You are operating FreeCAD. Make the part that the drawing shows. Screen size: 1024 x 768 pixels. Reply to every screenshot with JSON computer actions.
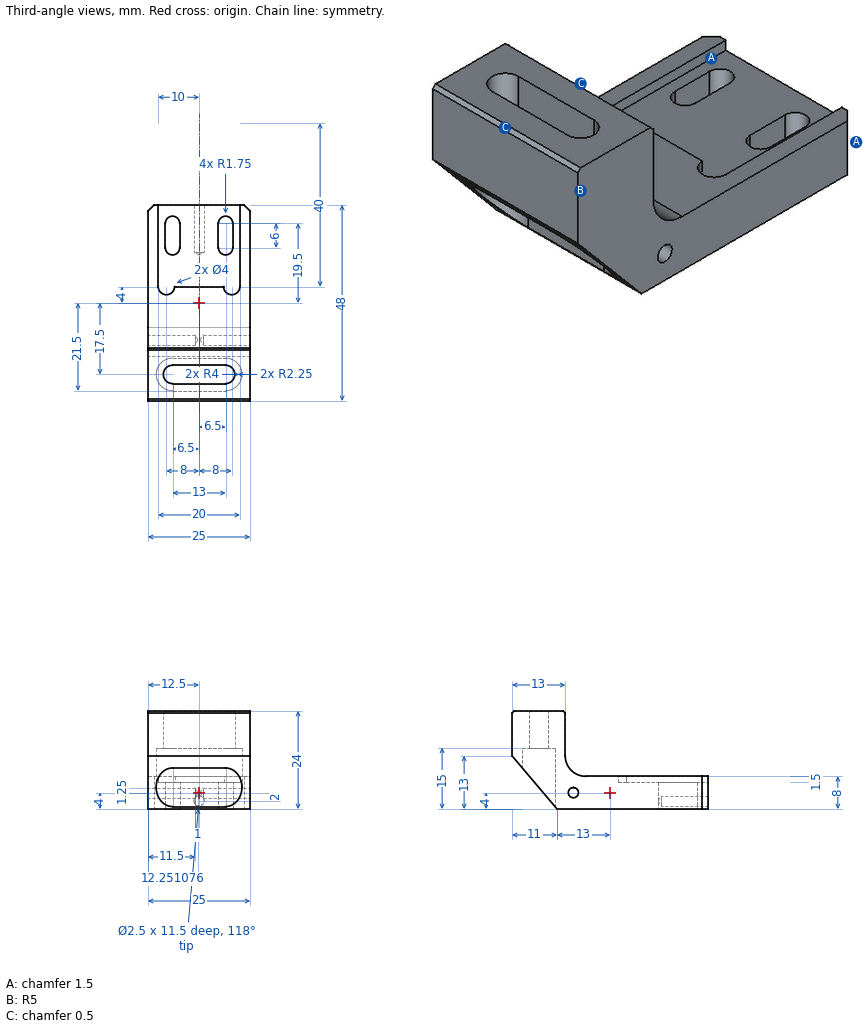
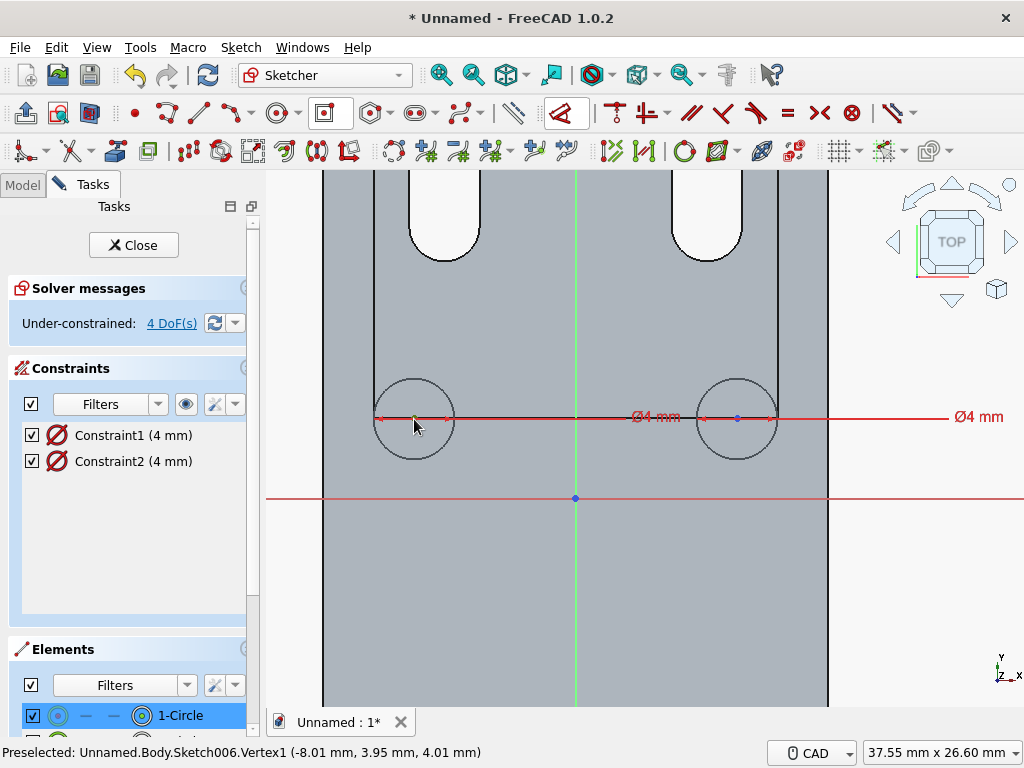
{"action": "left_click", "coordinate": [737, 419]}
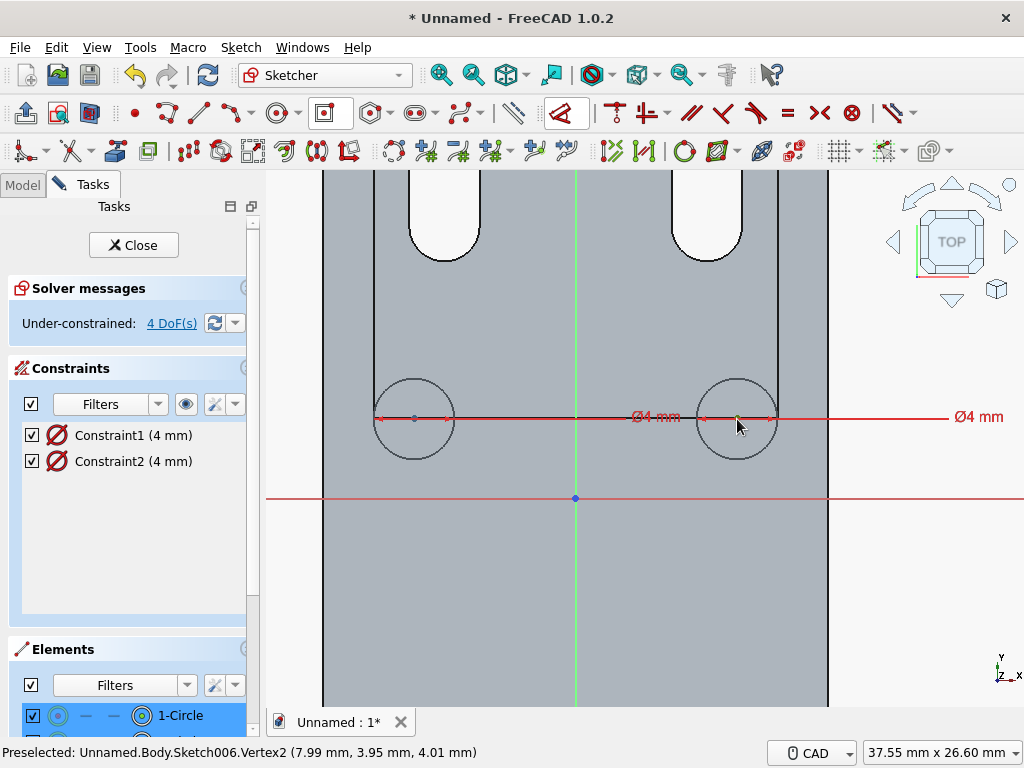
{"action": "left_click", "coordinate": [670, 114]}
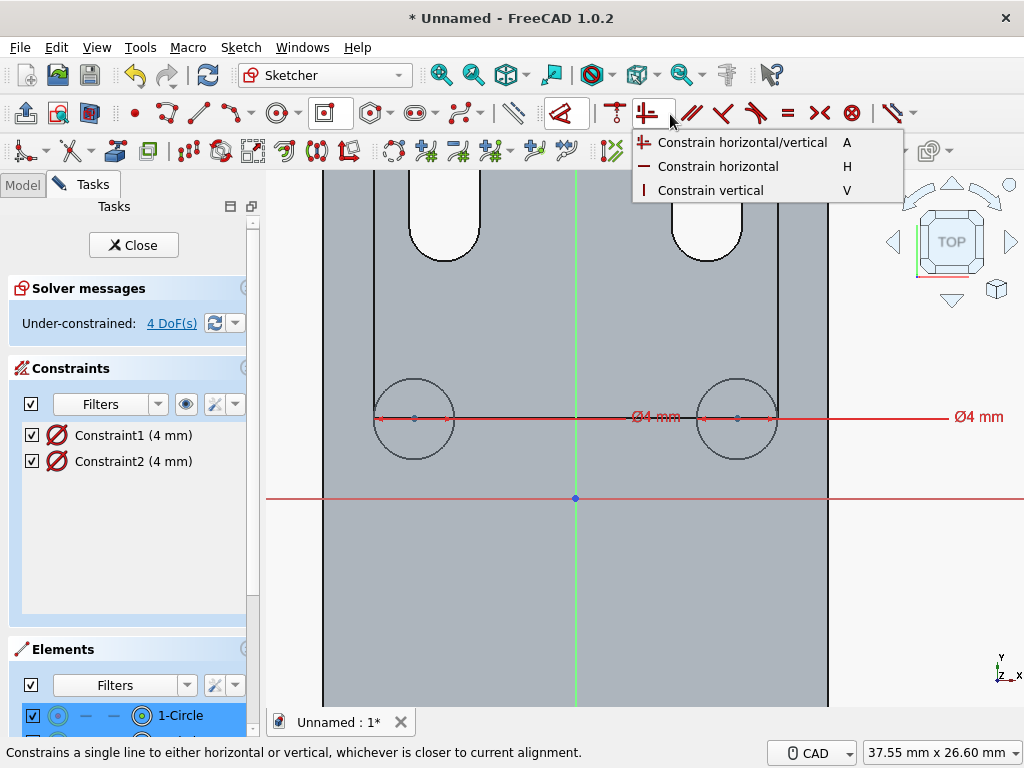
{"action": "left_click", "coordinate": [768, 166]}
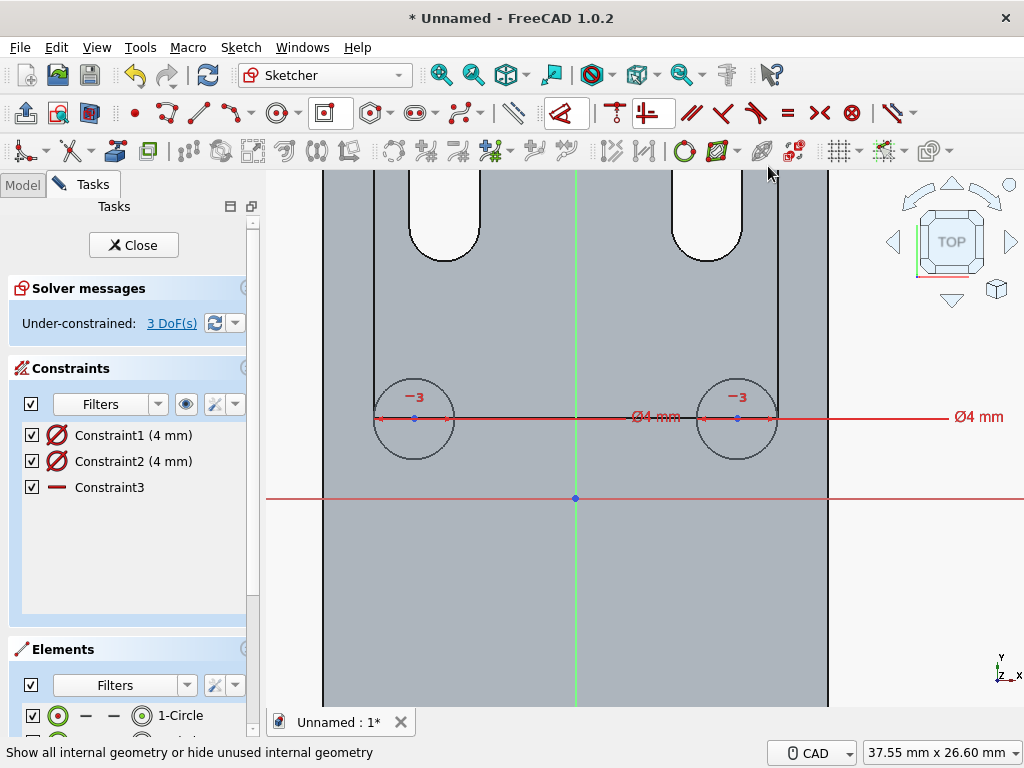
{"action": "left_click", "coordinate": [414, 419]}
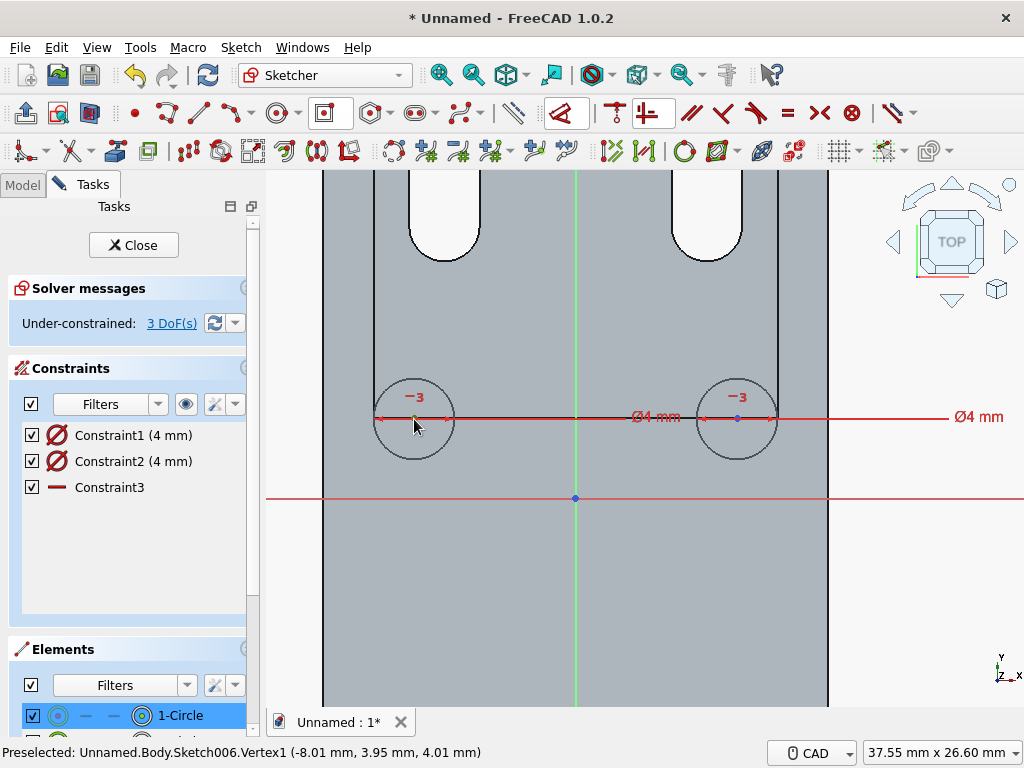
{"action": "left_click", "coordinate": [584, 114]}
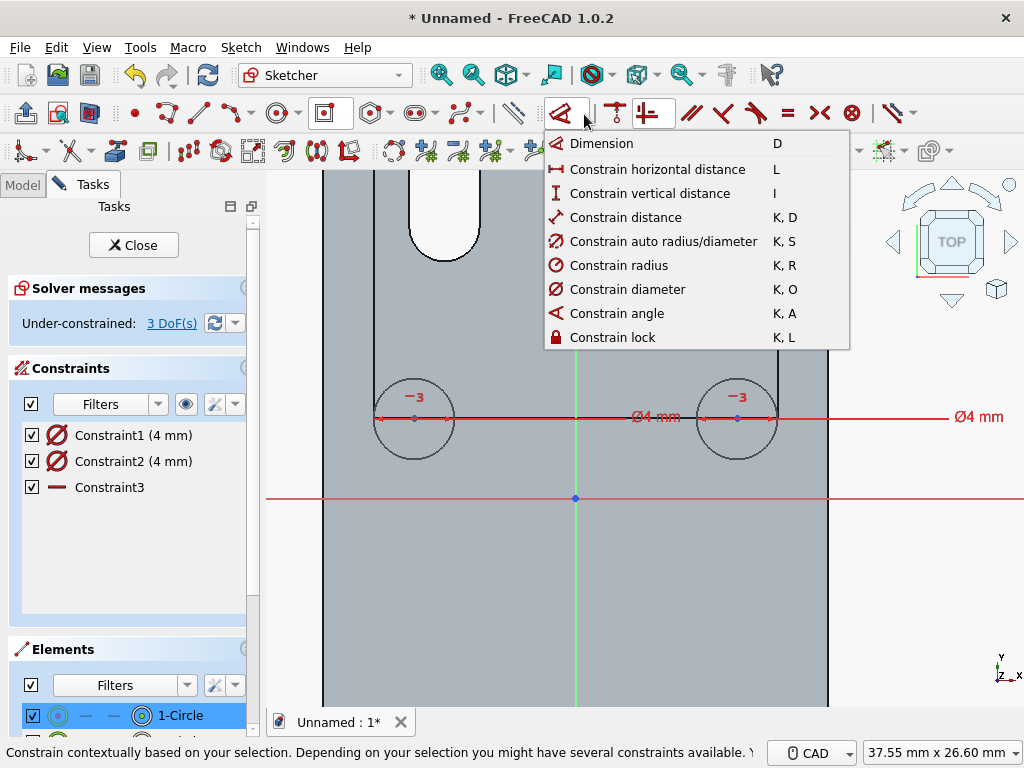
{"action": "left_click", "coordinate": [697, 169]}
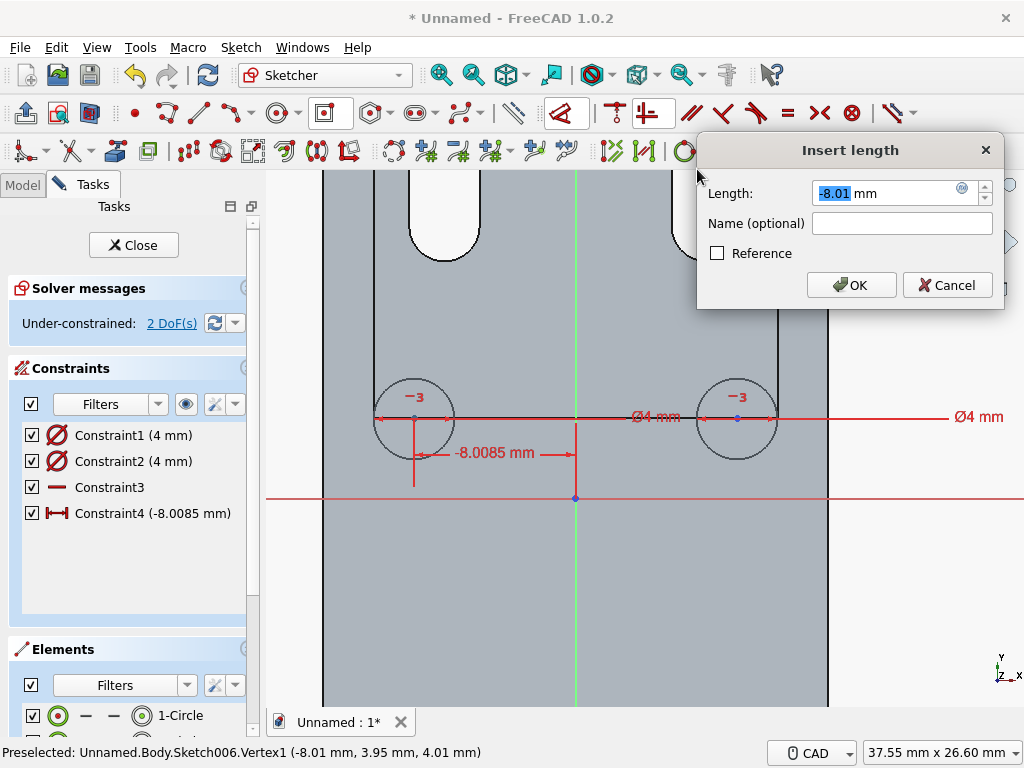
{"action": "type", "text": "-8"}
{"action": "key", "text": "Return"}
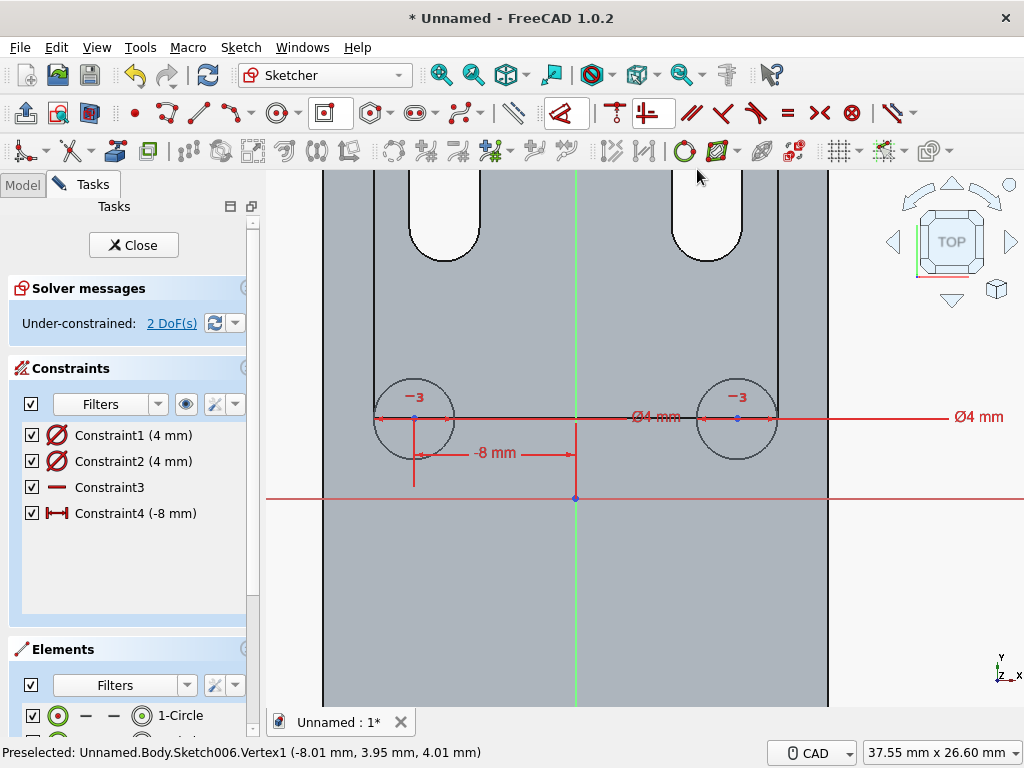
{"action": "left_click", "coordinate": [414, 419]}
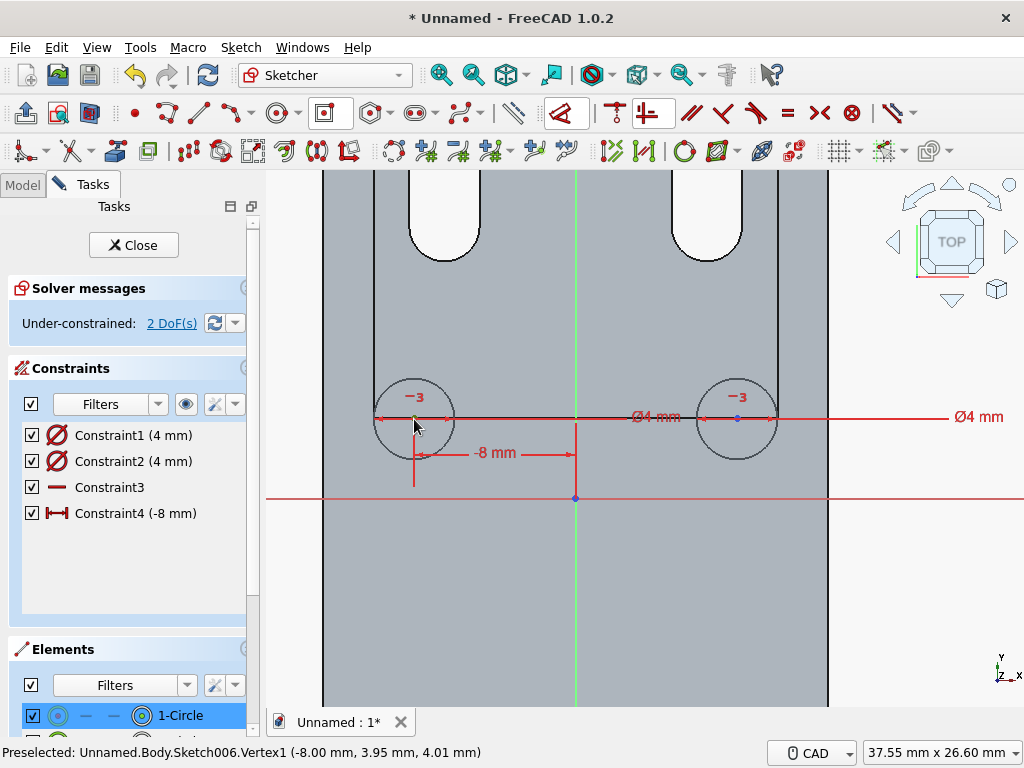
{"action": "left_click", "coordinate": [584, 114]}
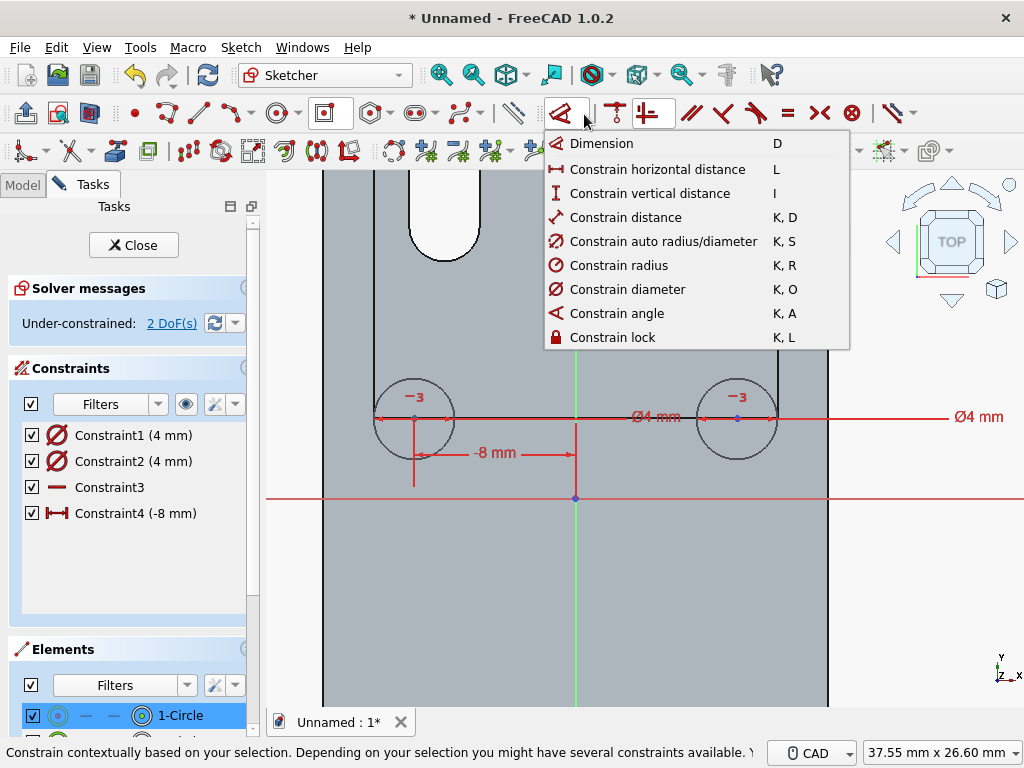
{"action": "left_click", "coordinate": [697, 193]}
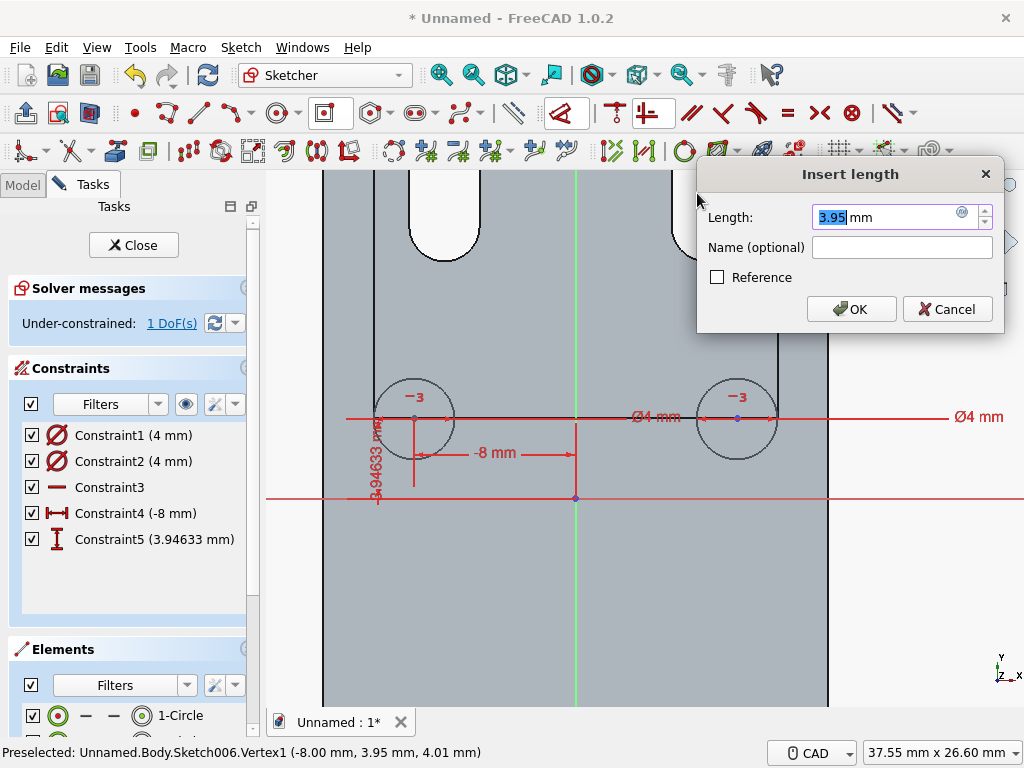
{"action": "type", "text": "4"}
{"action": "key", "text": "Return"}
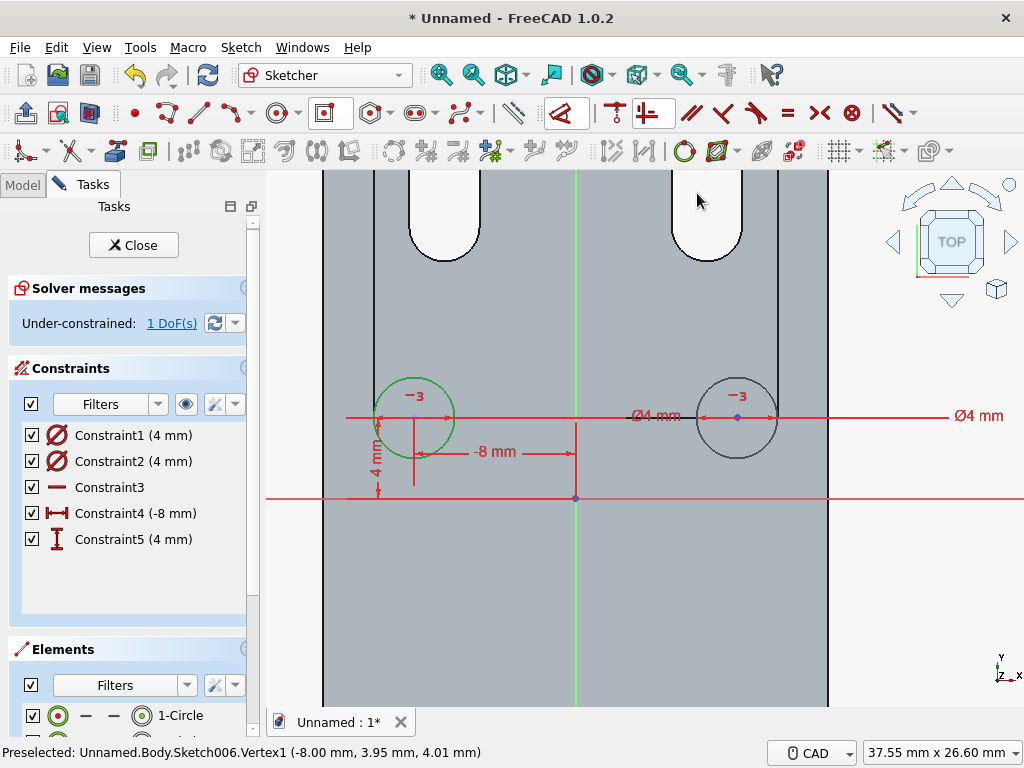
{"action": "left_click", "coordinate": [737, 418]}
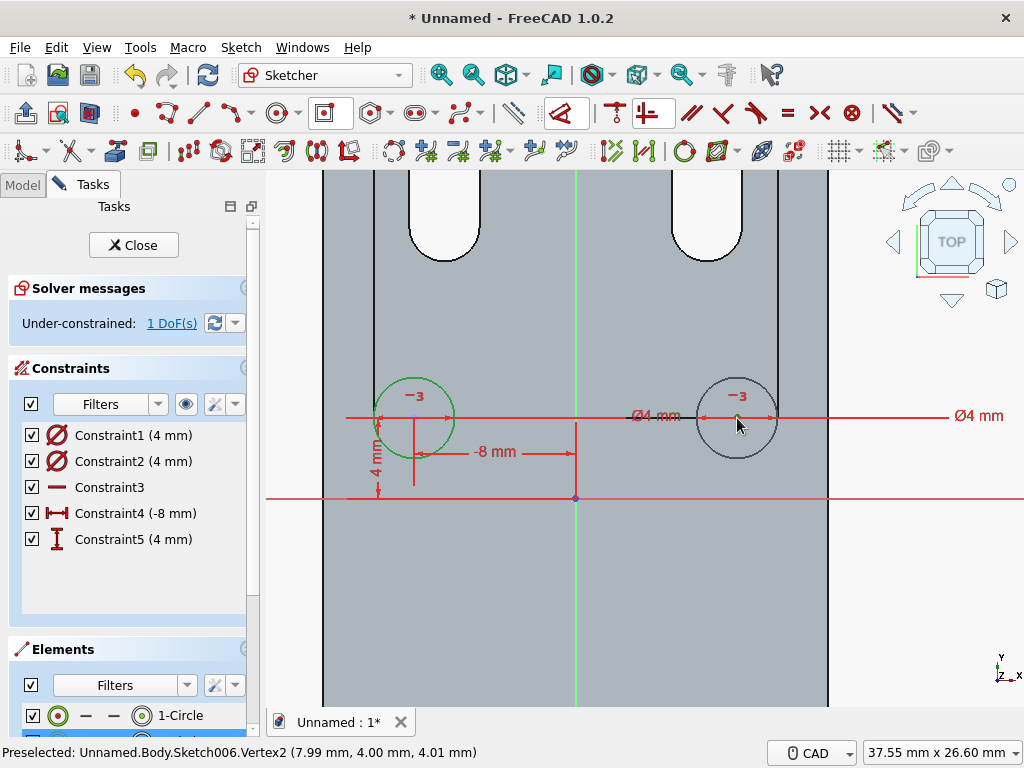
{"action": "key", "text": "l"}